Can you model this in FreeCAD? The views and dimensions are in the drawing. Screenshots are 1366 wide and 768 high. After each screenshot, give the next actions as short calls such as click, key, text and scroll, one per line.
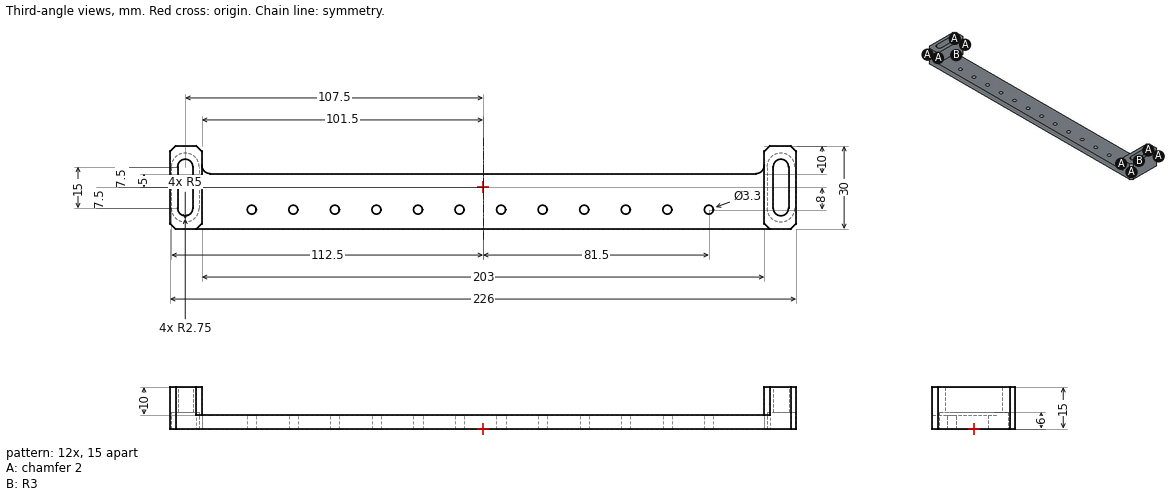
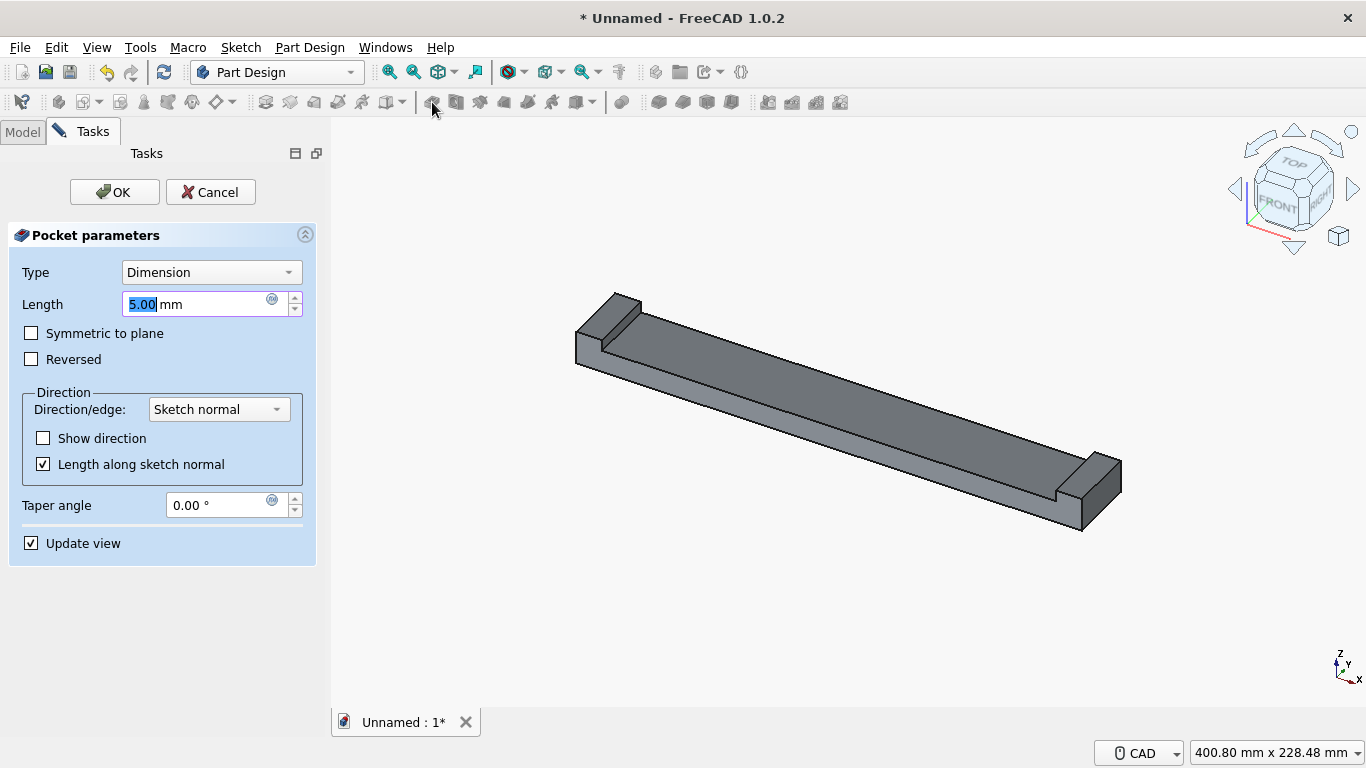
text(10)
key(Tab)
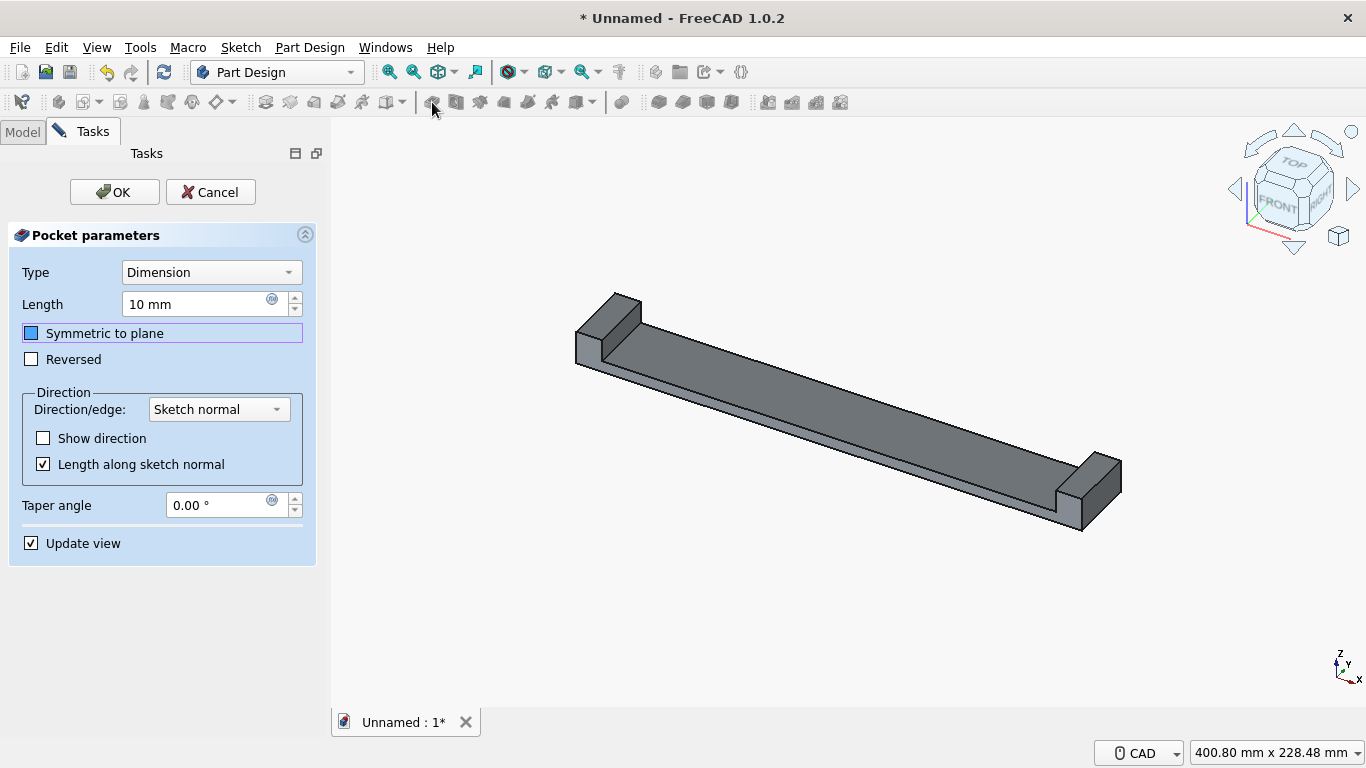
click(115, 192)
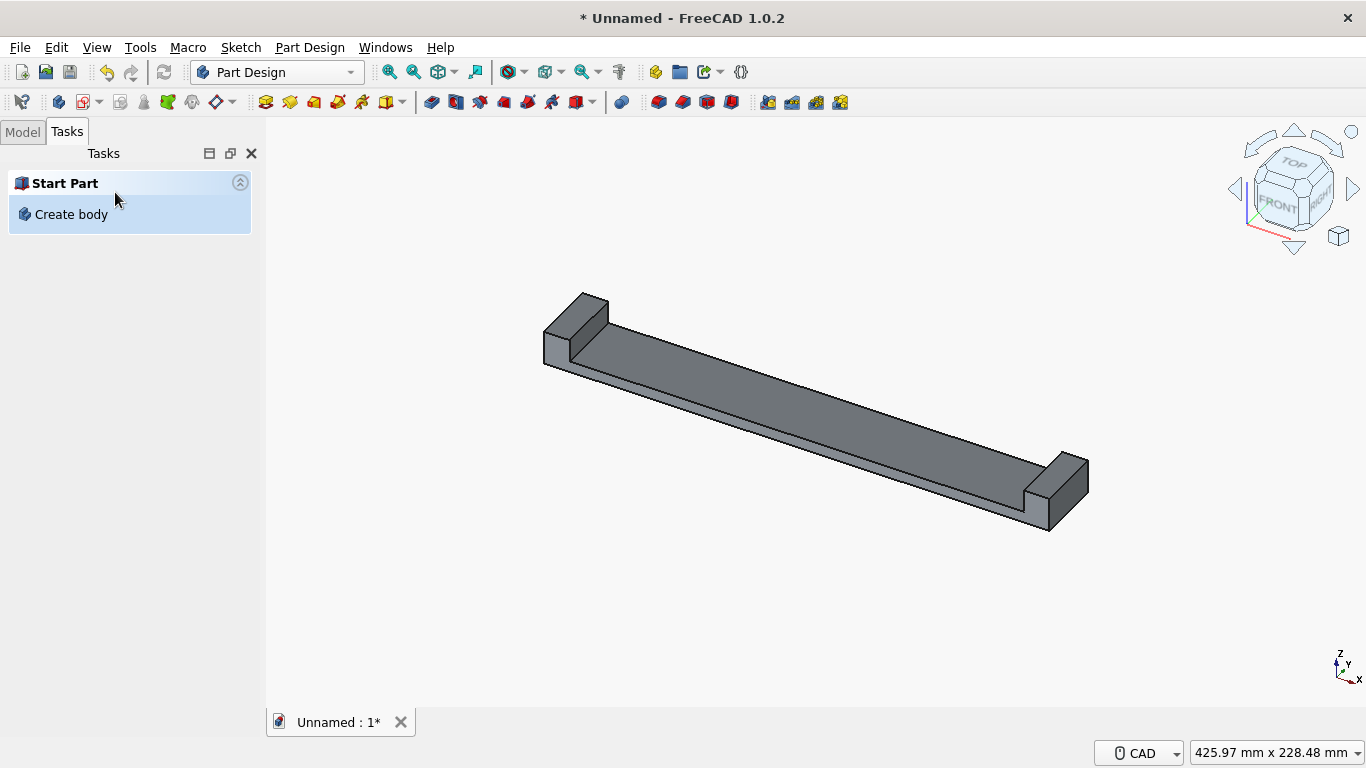
click(946, 459)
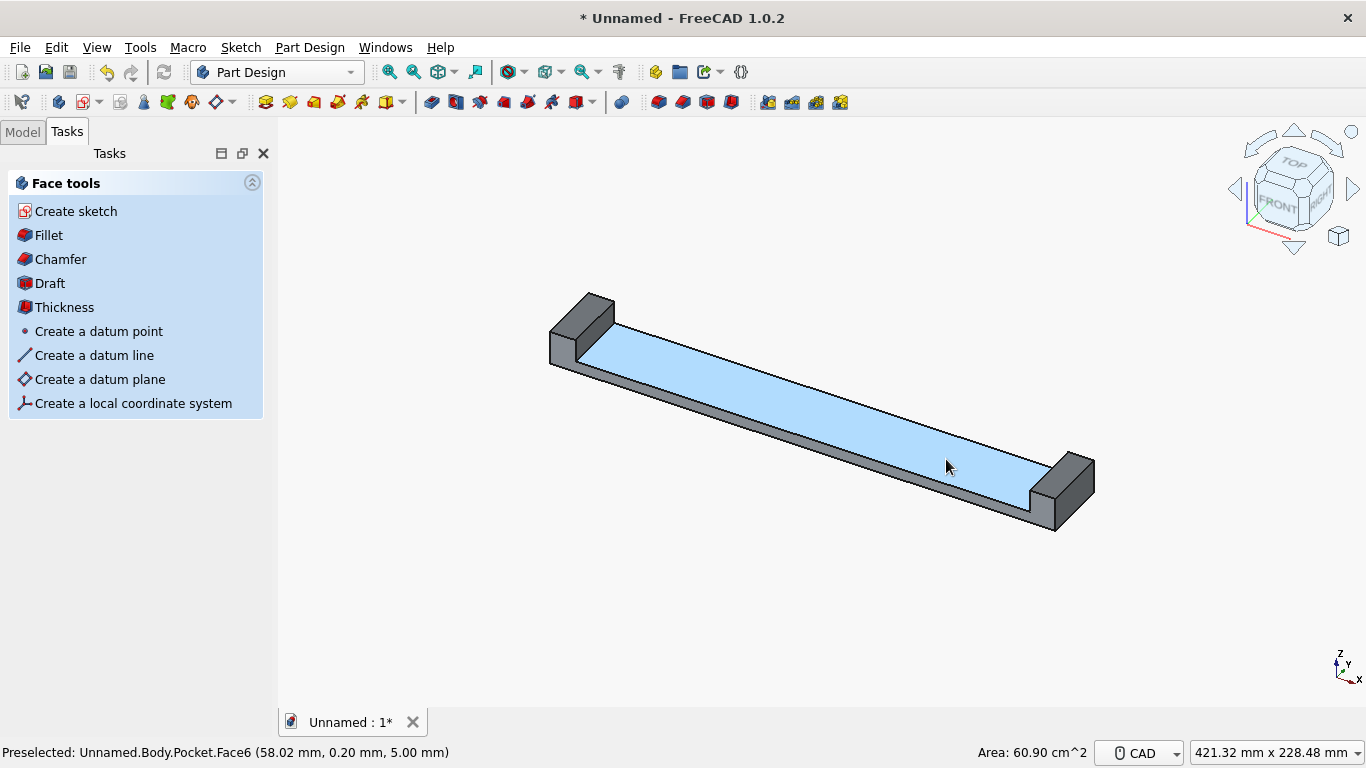
click(84, 102)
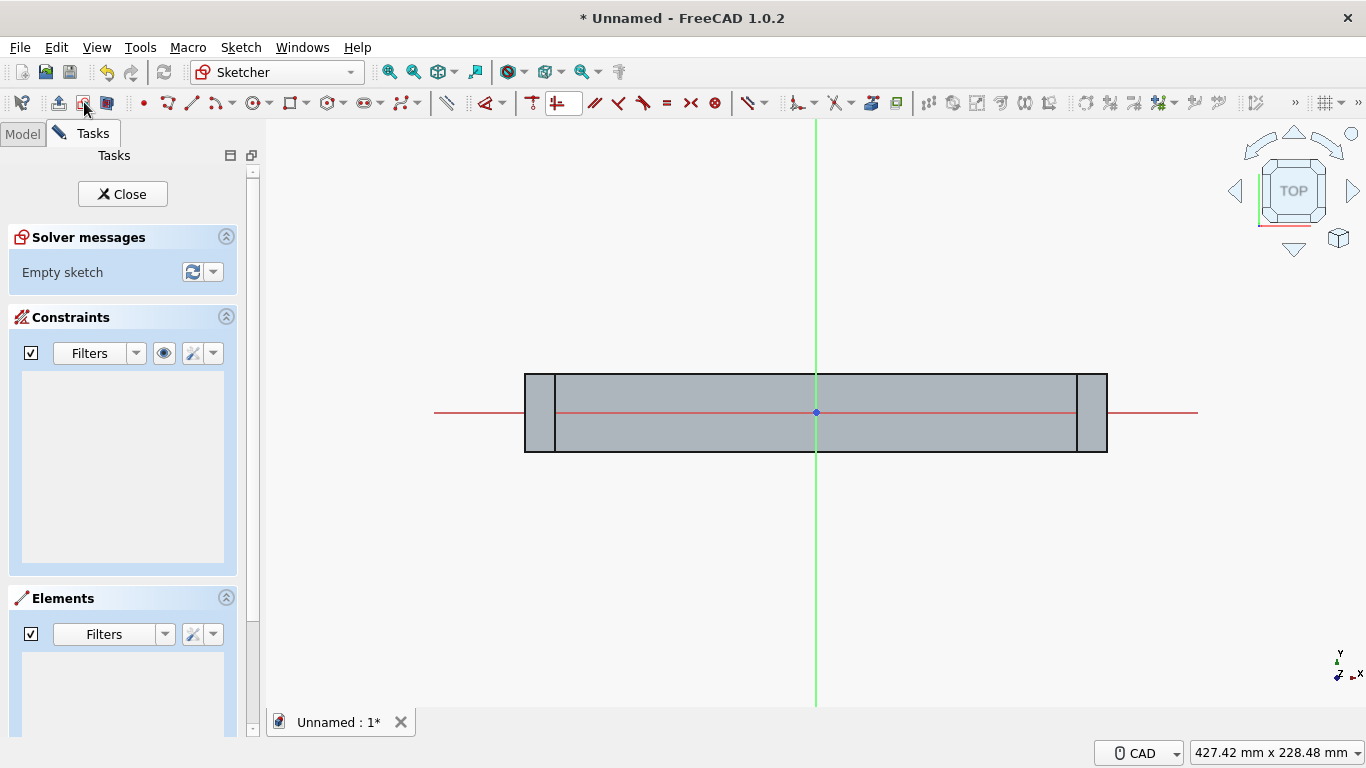
click(290, 104)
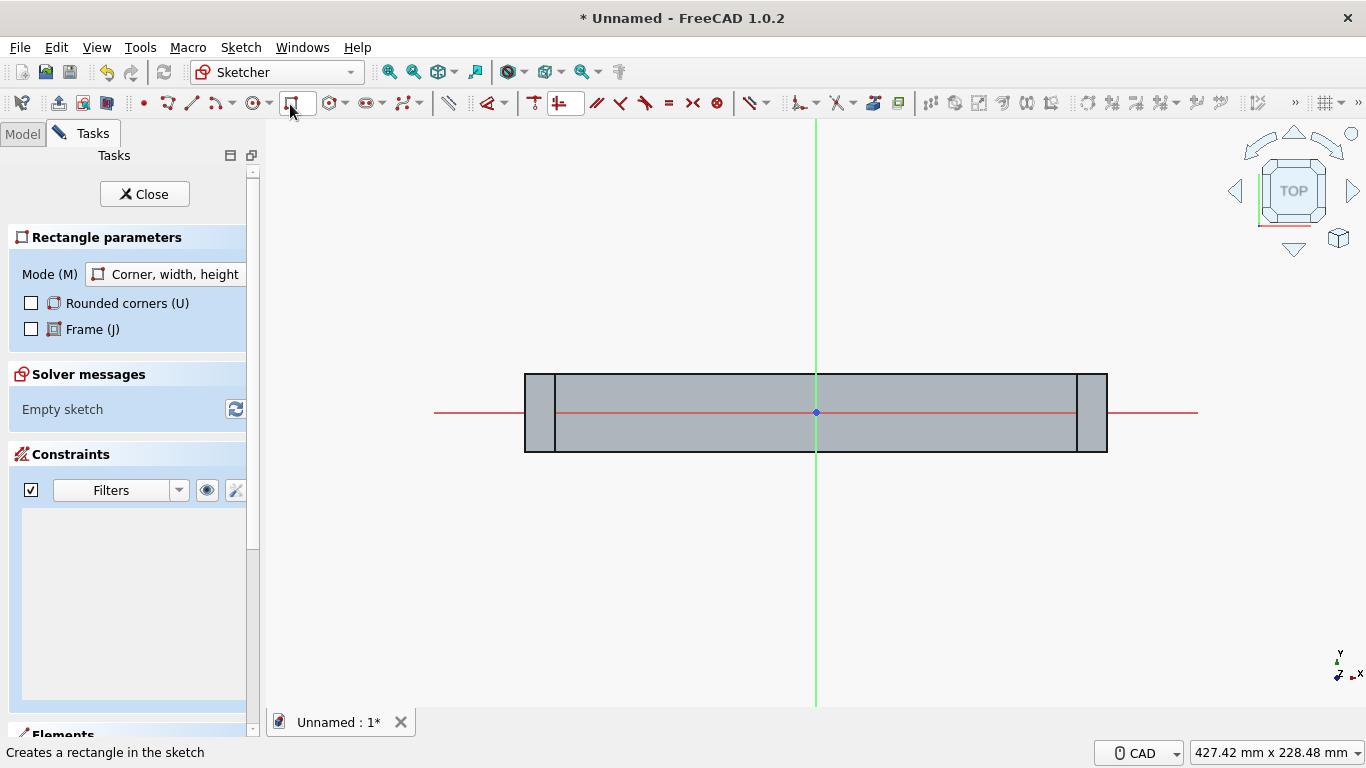
click(555, 374)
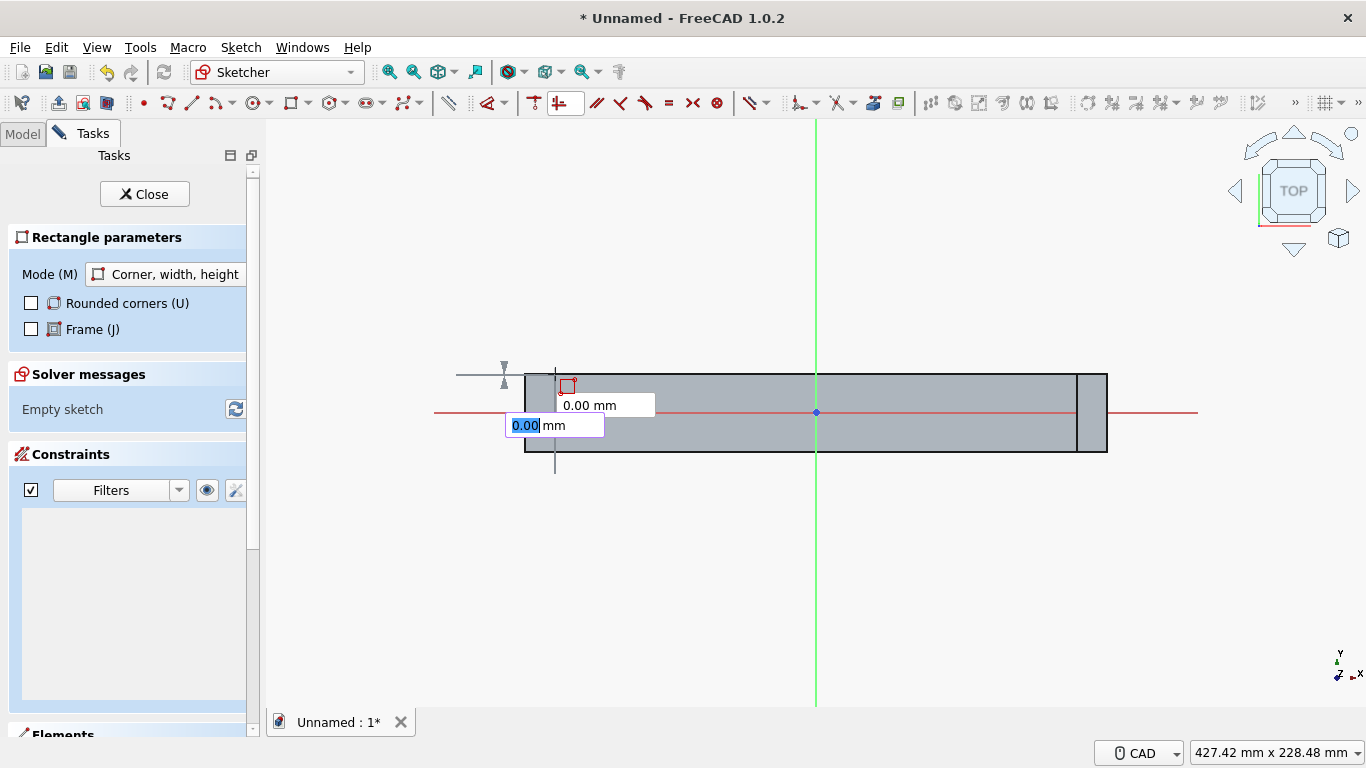
scroll(1077, 400, up, 2)
move(1077, 400)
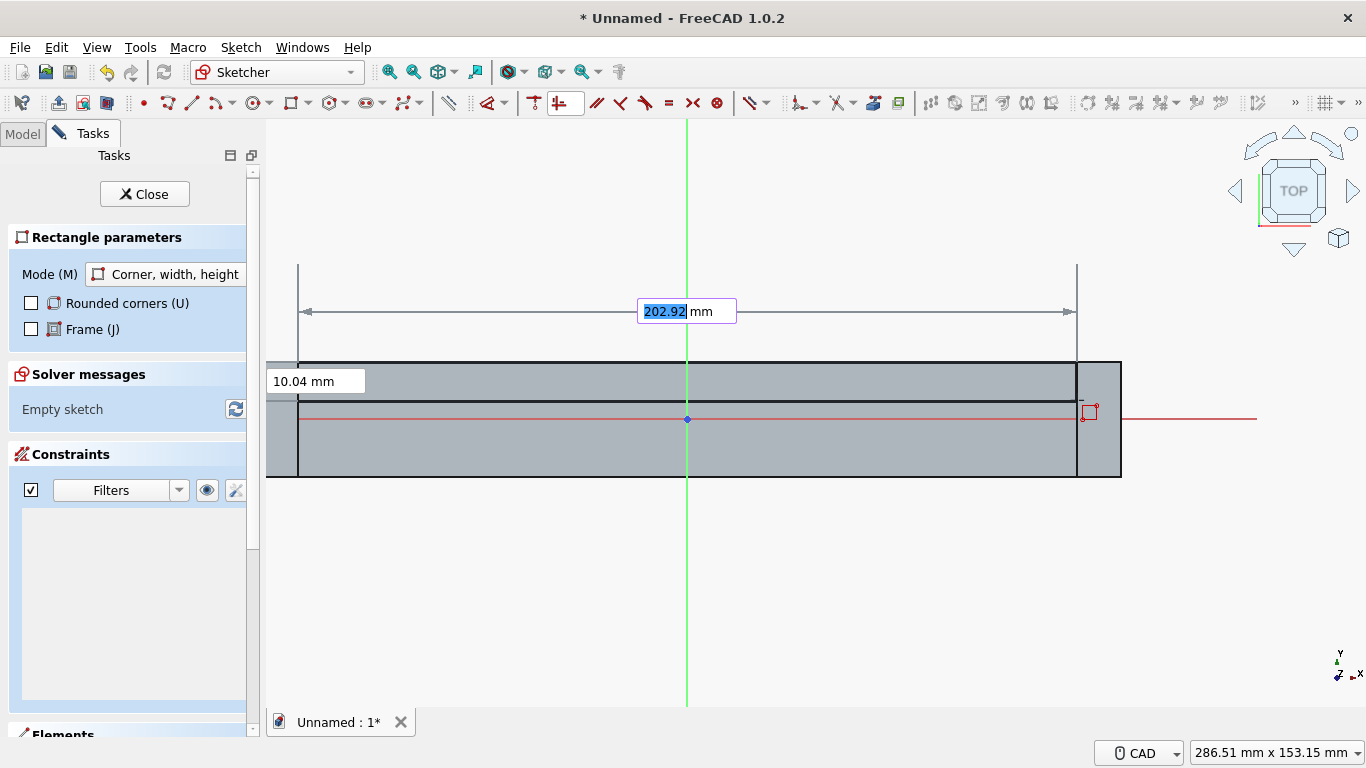
text(203)
key(Tab)
text(10)
key(Return)
key(Escape)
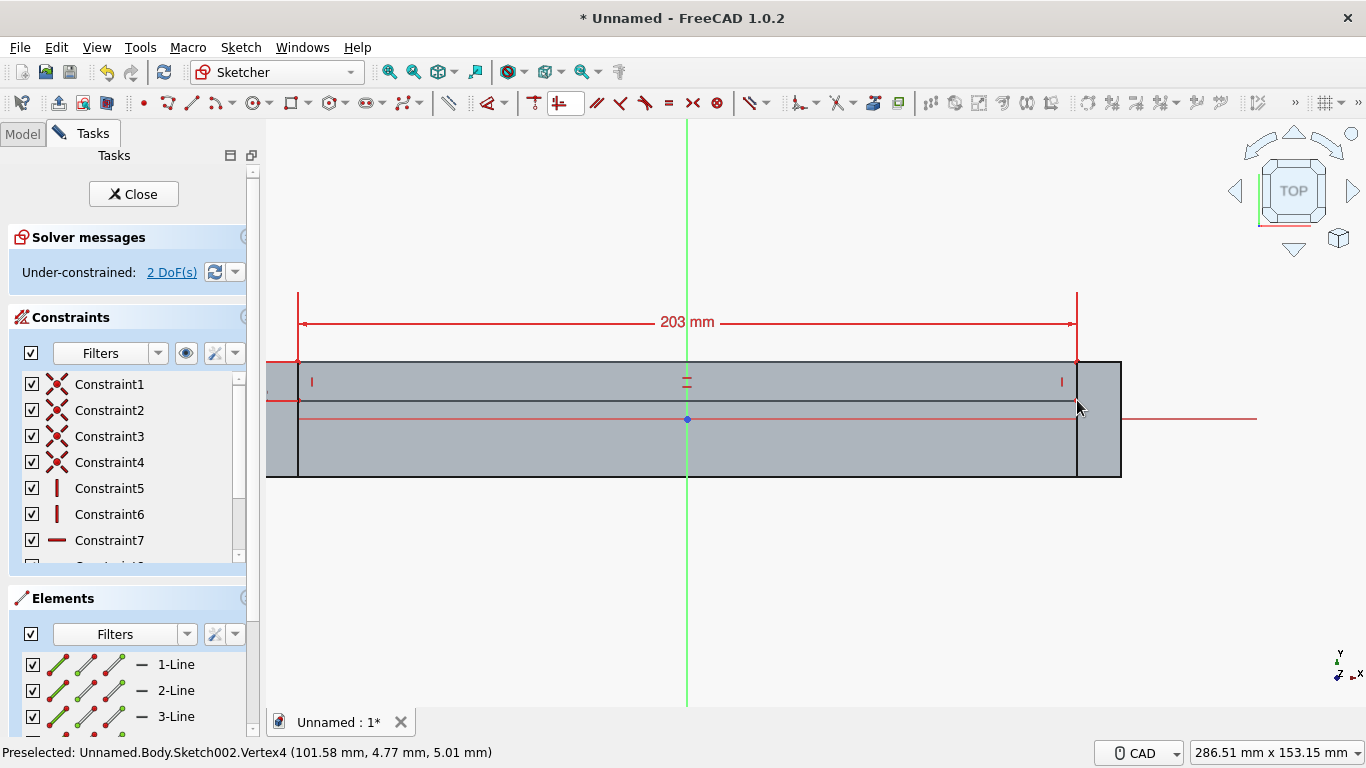
key(d)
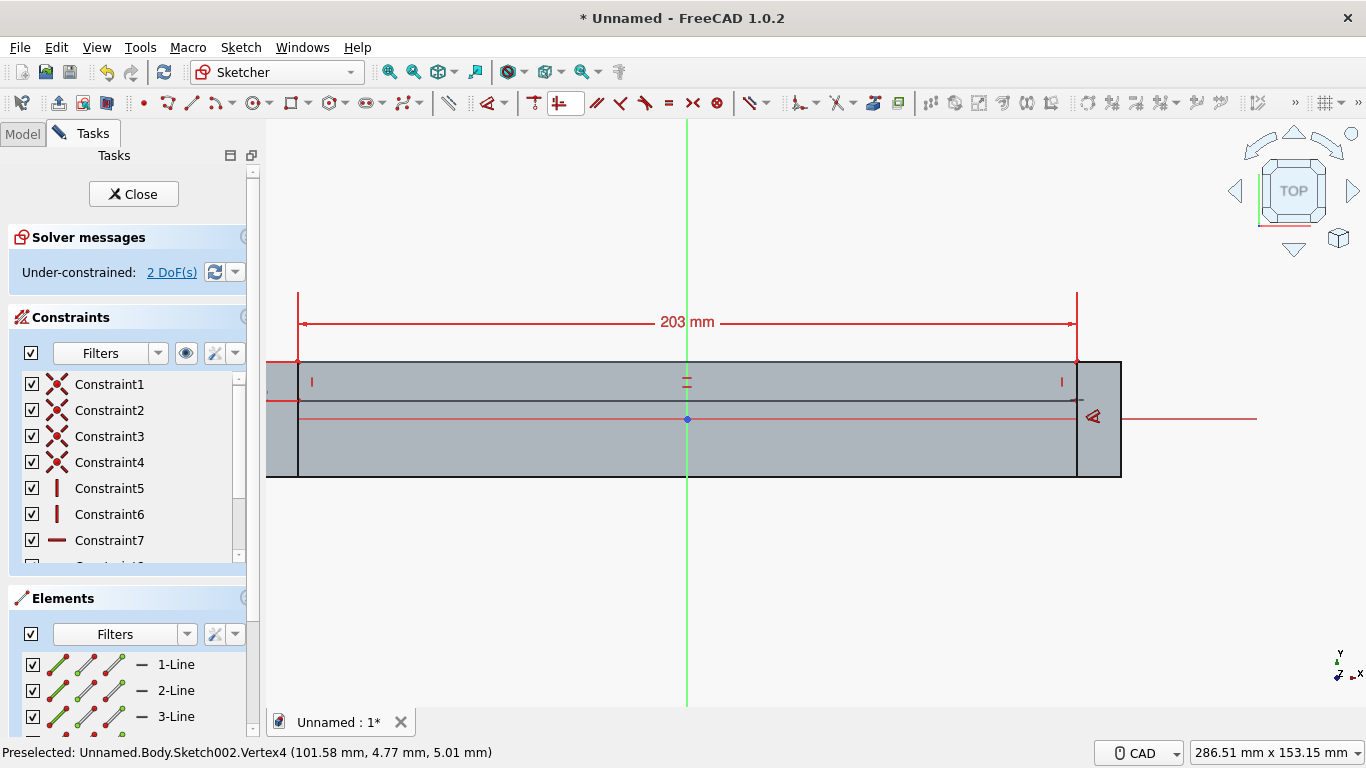
scroll(298, 401, up, 4)